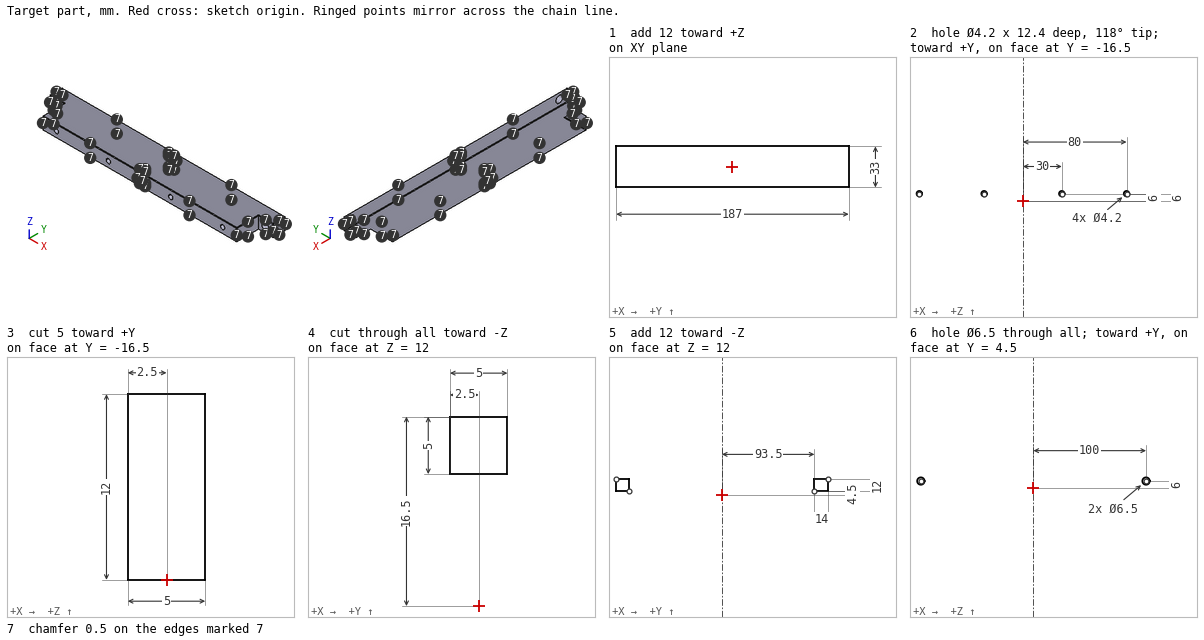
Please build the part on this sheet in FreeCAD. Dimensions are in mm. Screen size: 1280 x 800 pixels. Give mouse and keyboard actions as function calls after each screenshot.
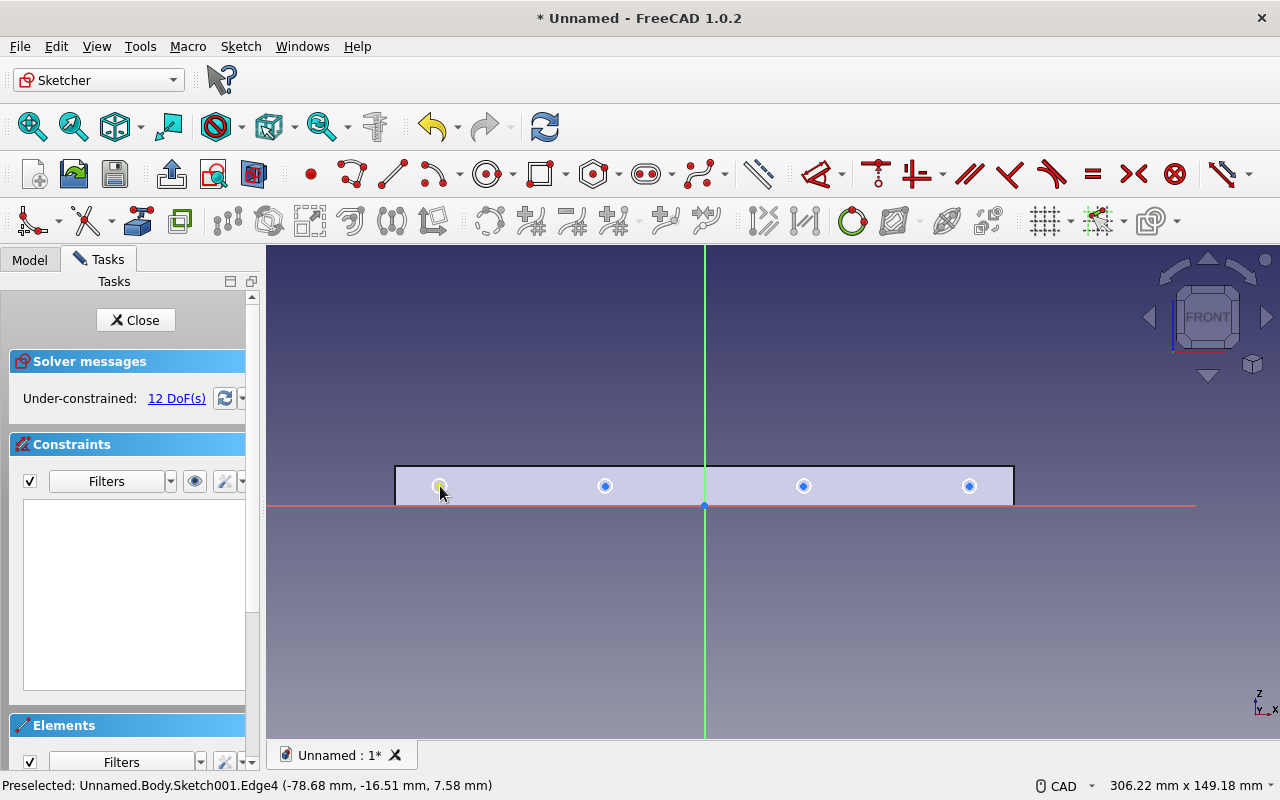
scroll(974, 481, up, 4)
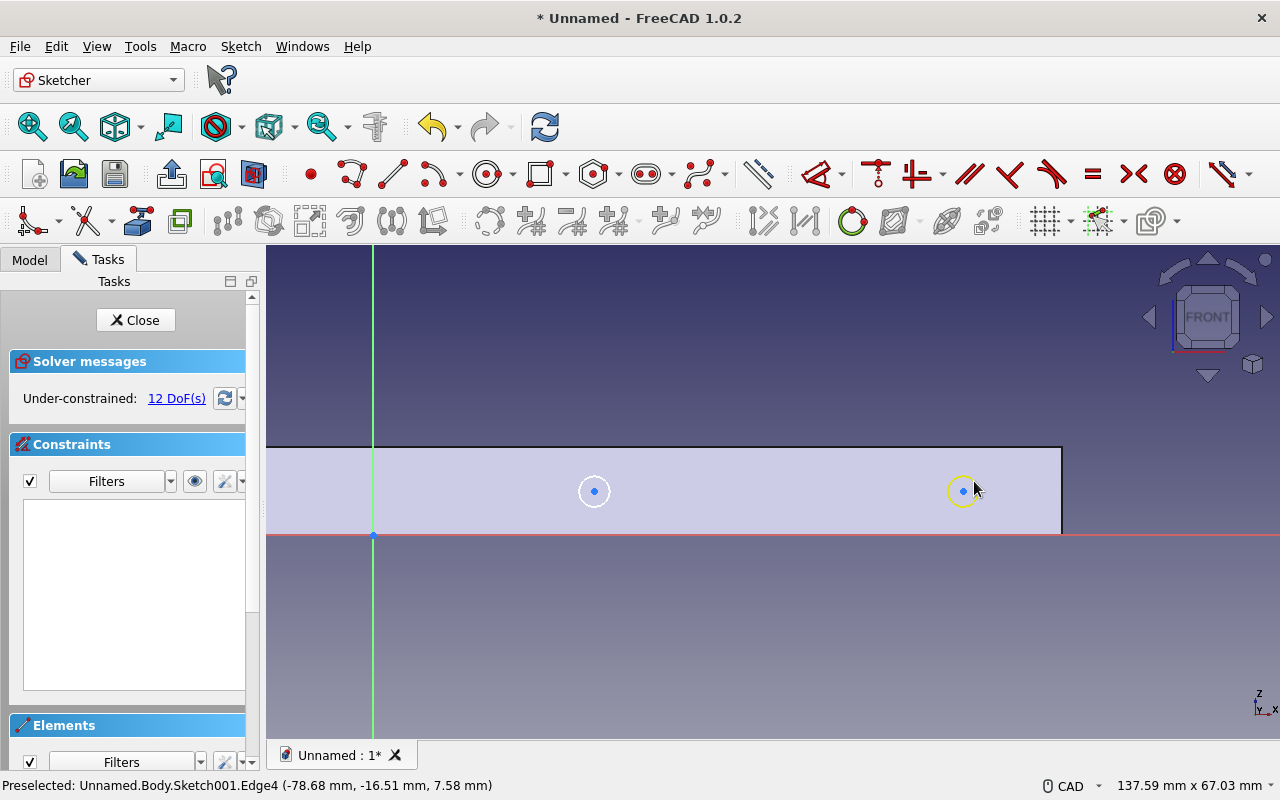
click(974, 481)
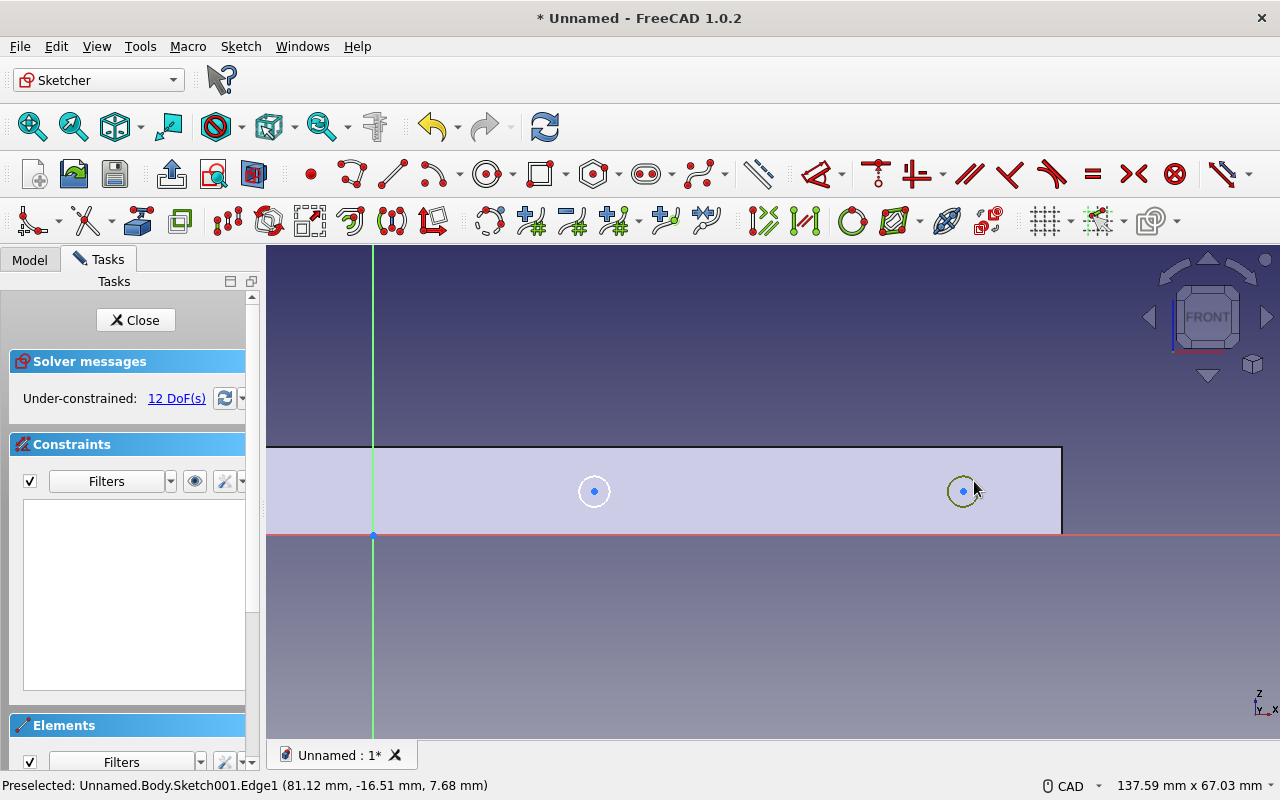
click(605, 481)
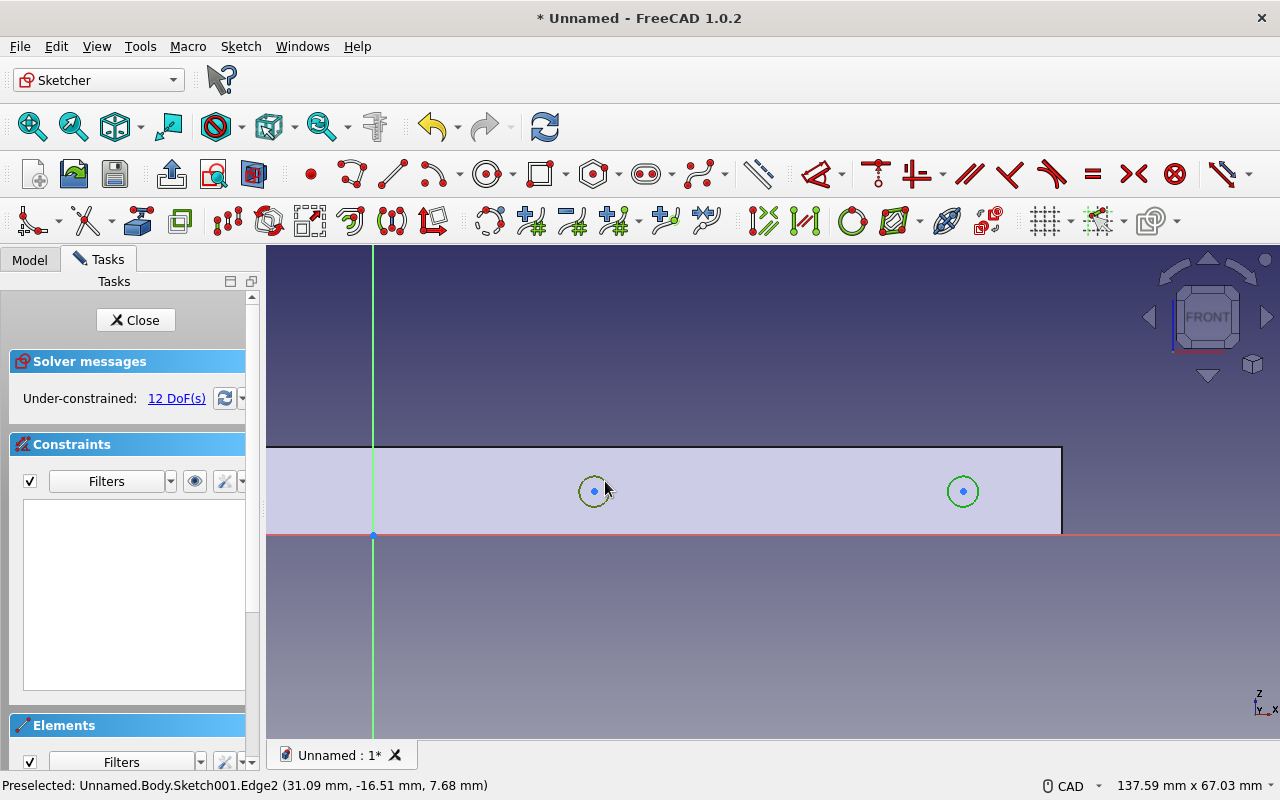
scroll(975, 481, down, 4)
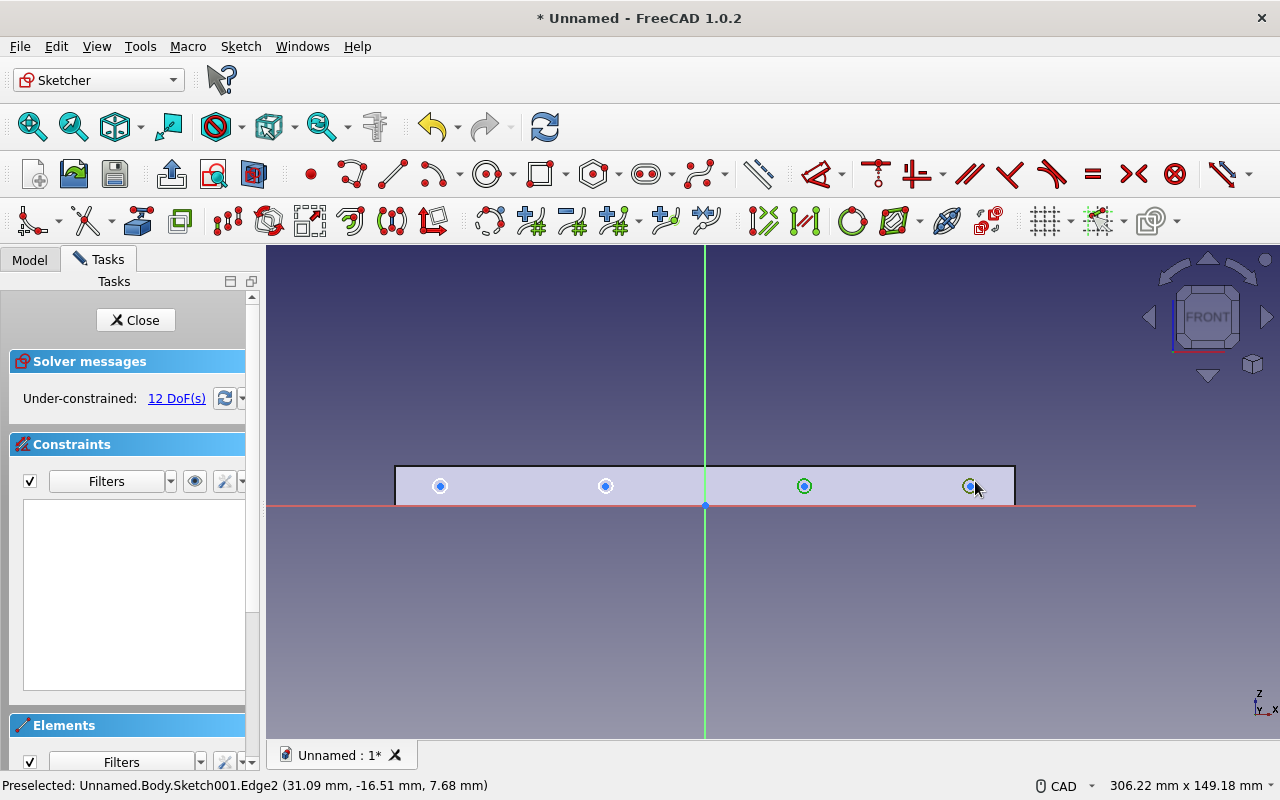
scroll(611, 481, up, 4)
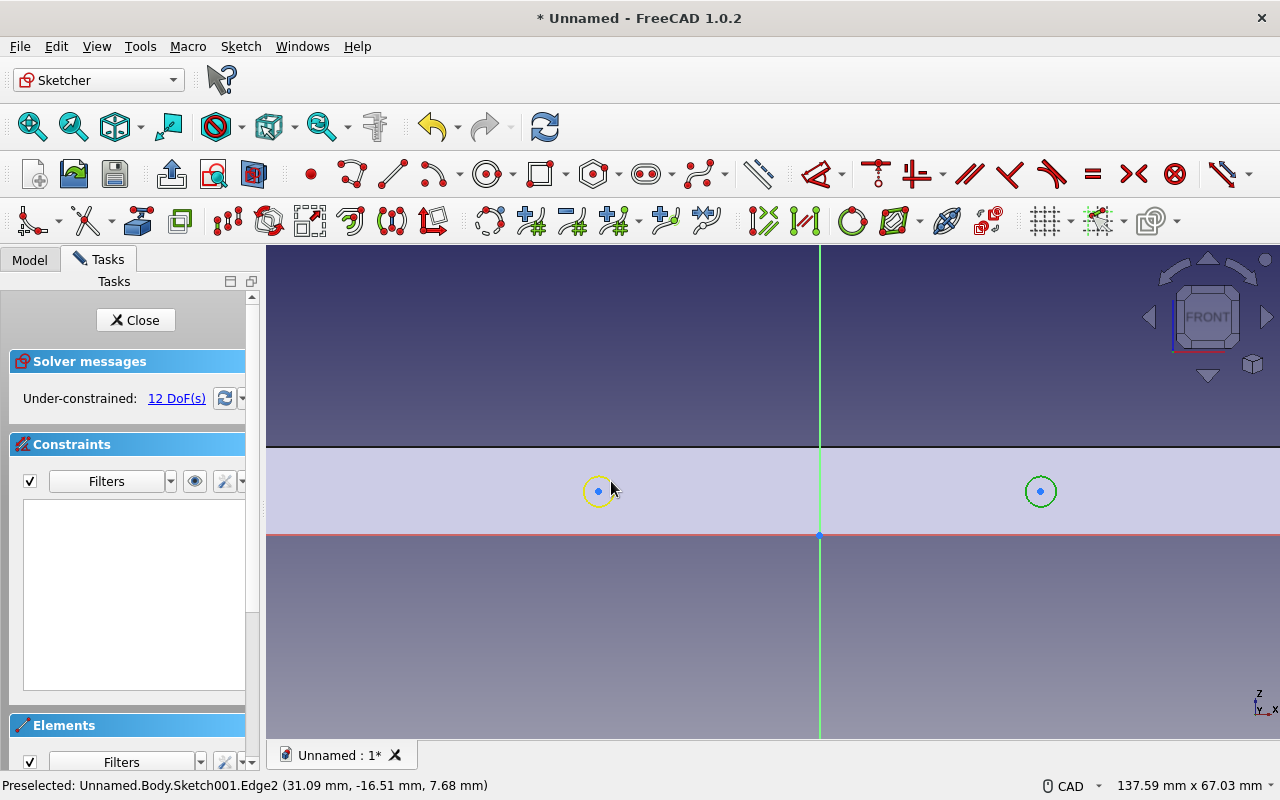
click(610, 481)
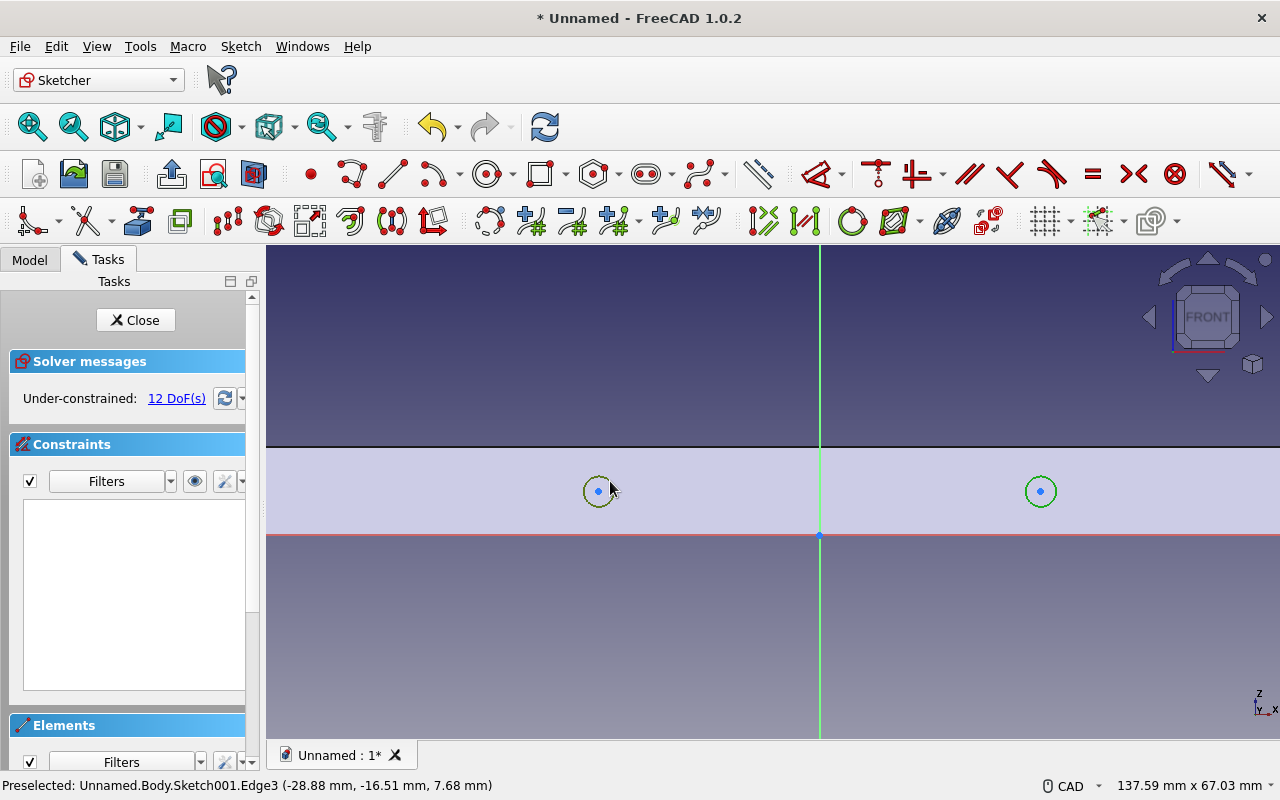
scroll(610, 481, down, 4)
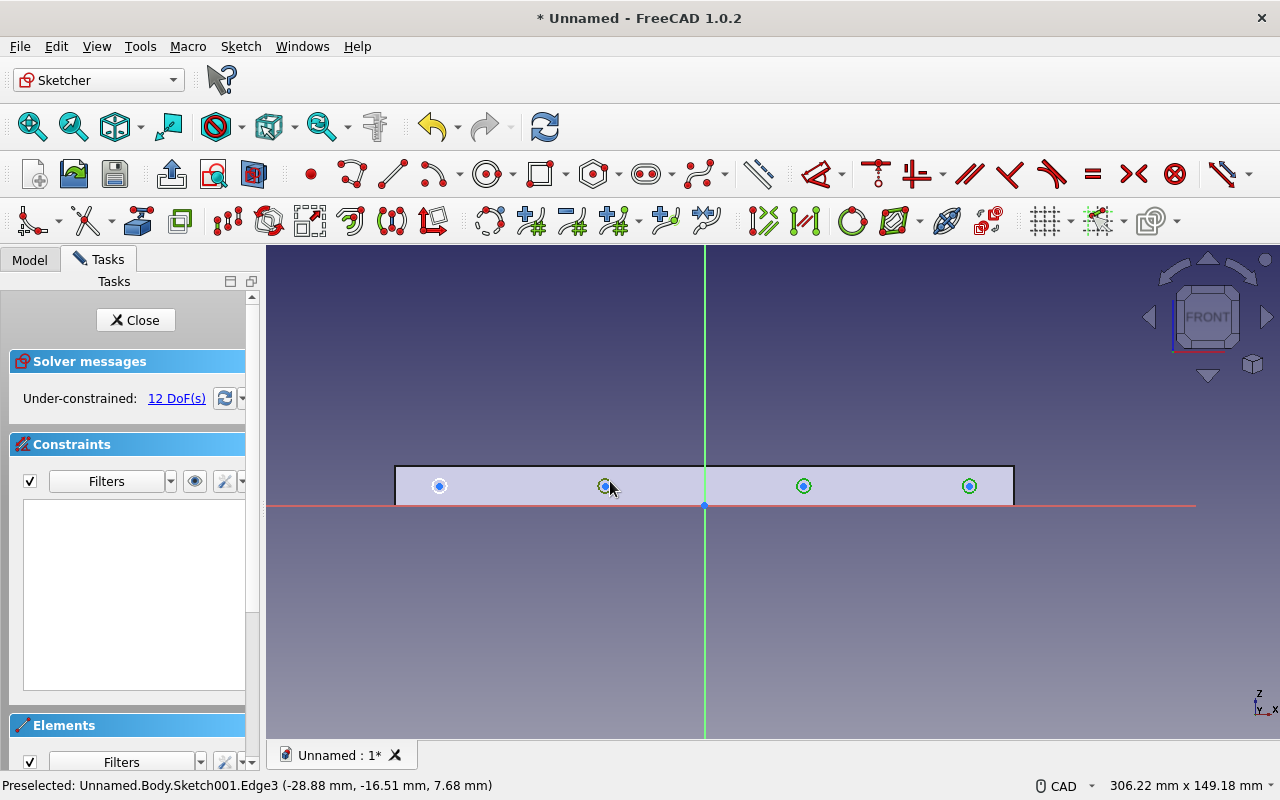
scroll(444, 481, up, 4)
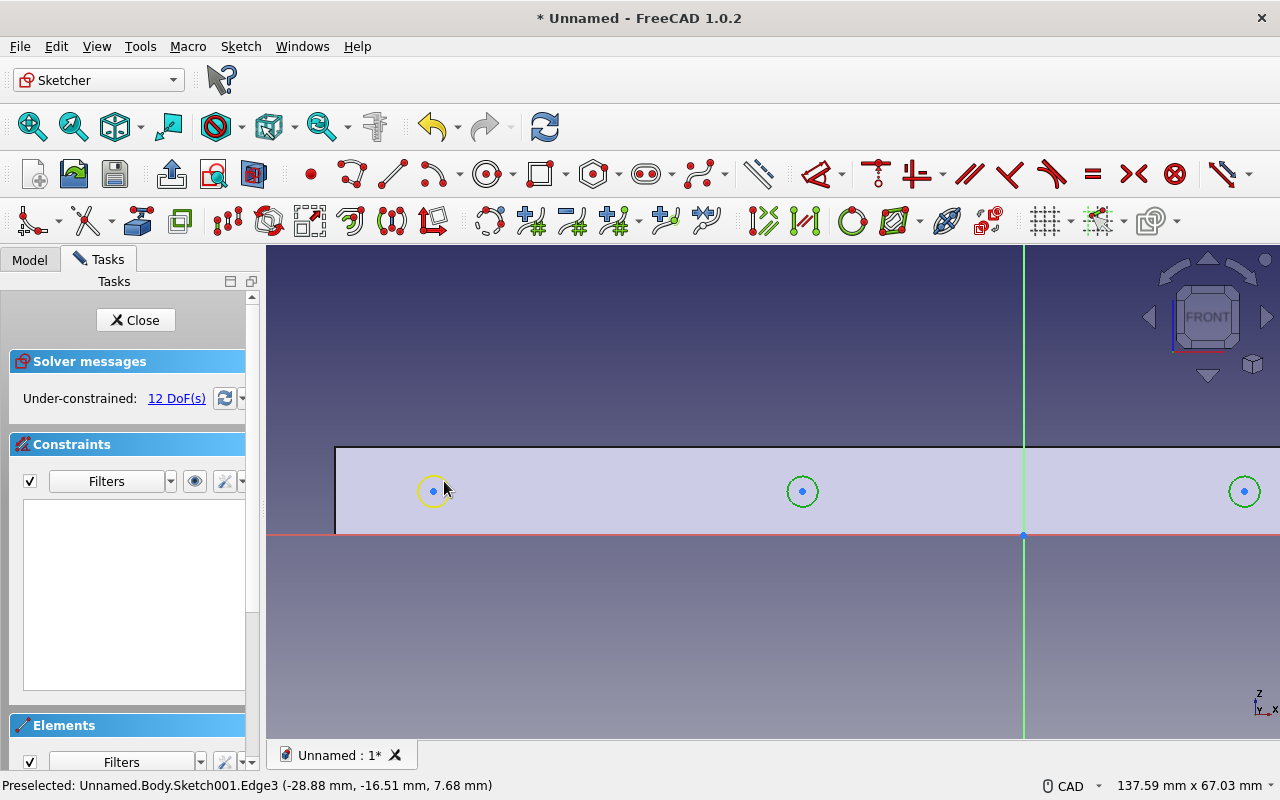
click(445, 481)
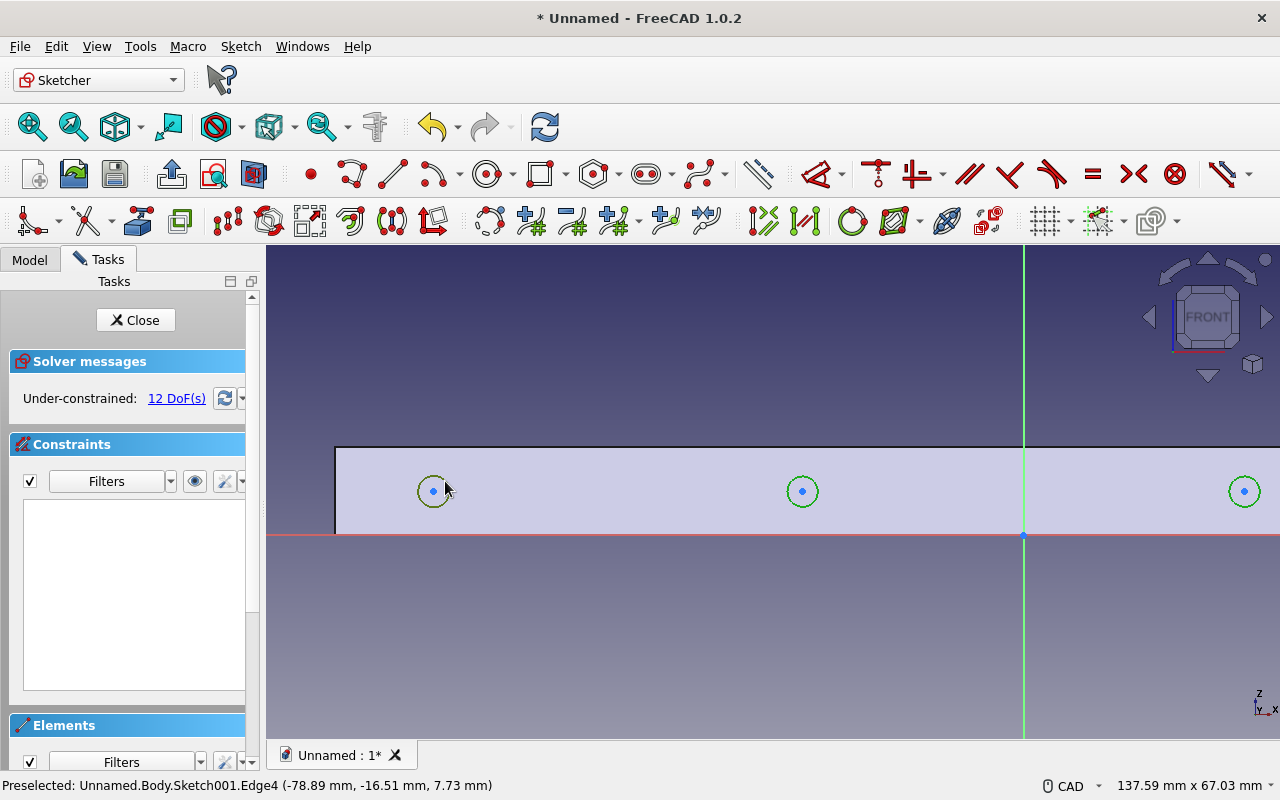
key(e)